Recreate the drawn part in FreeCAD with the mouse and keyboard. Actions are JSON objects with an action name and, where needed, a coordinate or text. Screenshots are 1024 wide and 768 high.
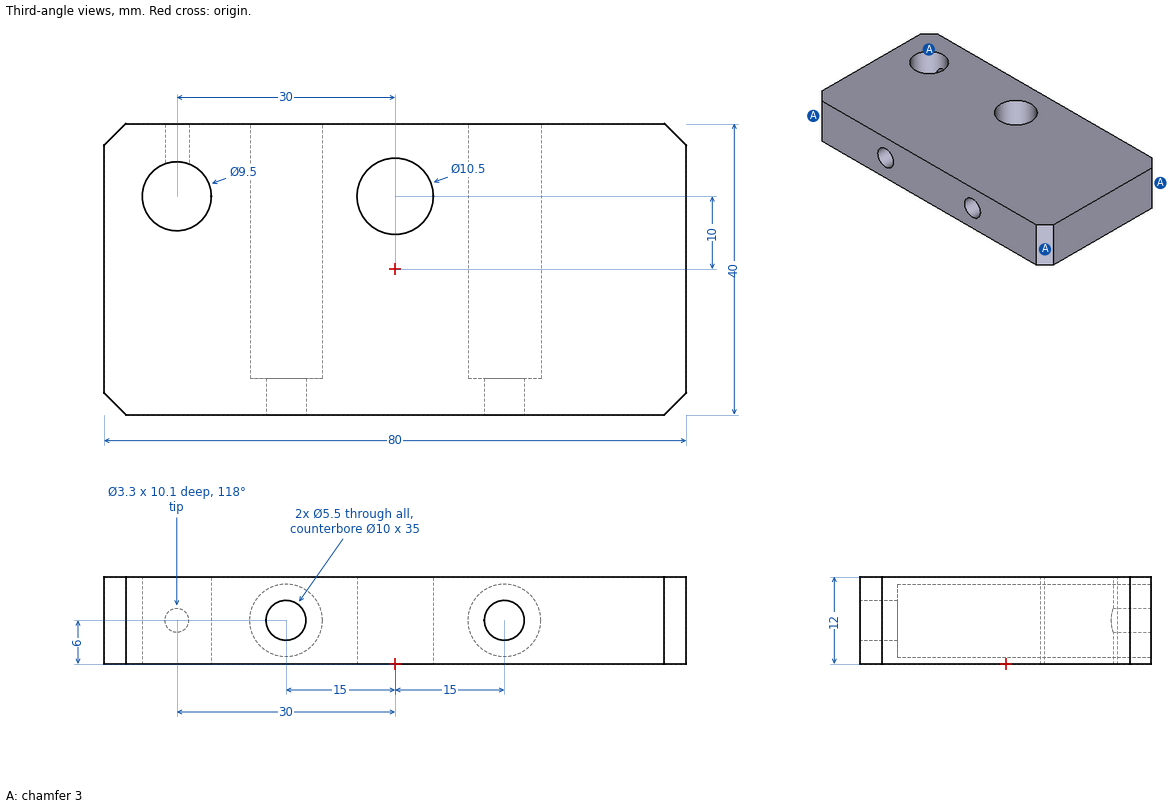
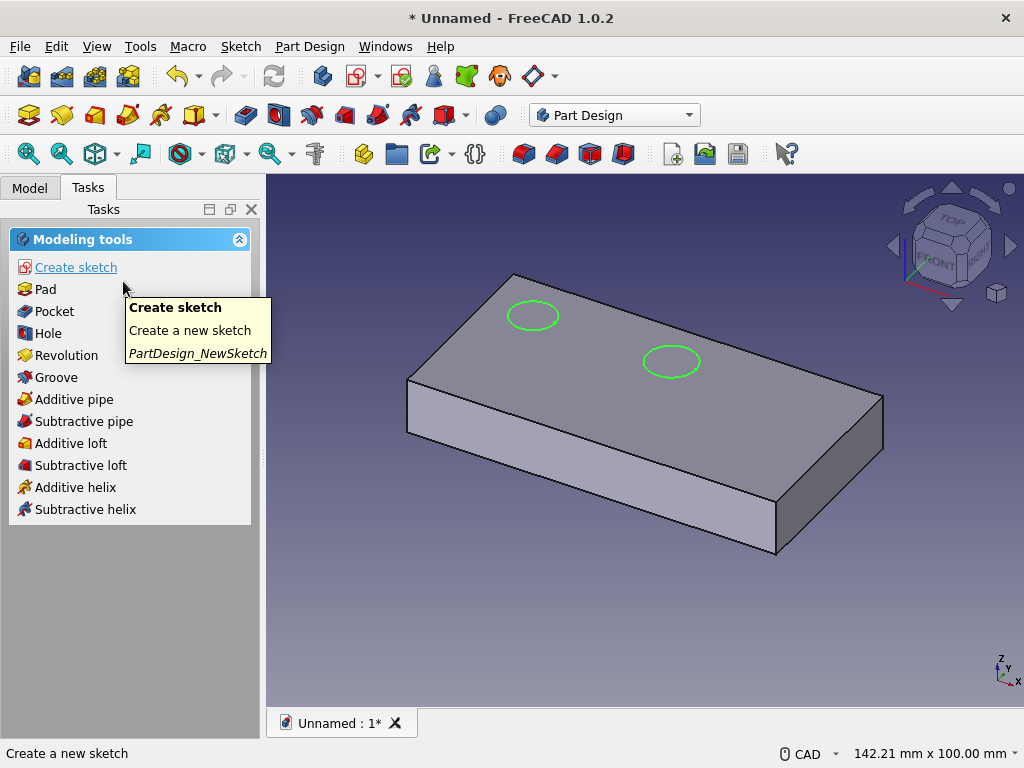
{"action": "left_click", "coordinate": [246, 116]}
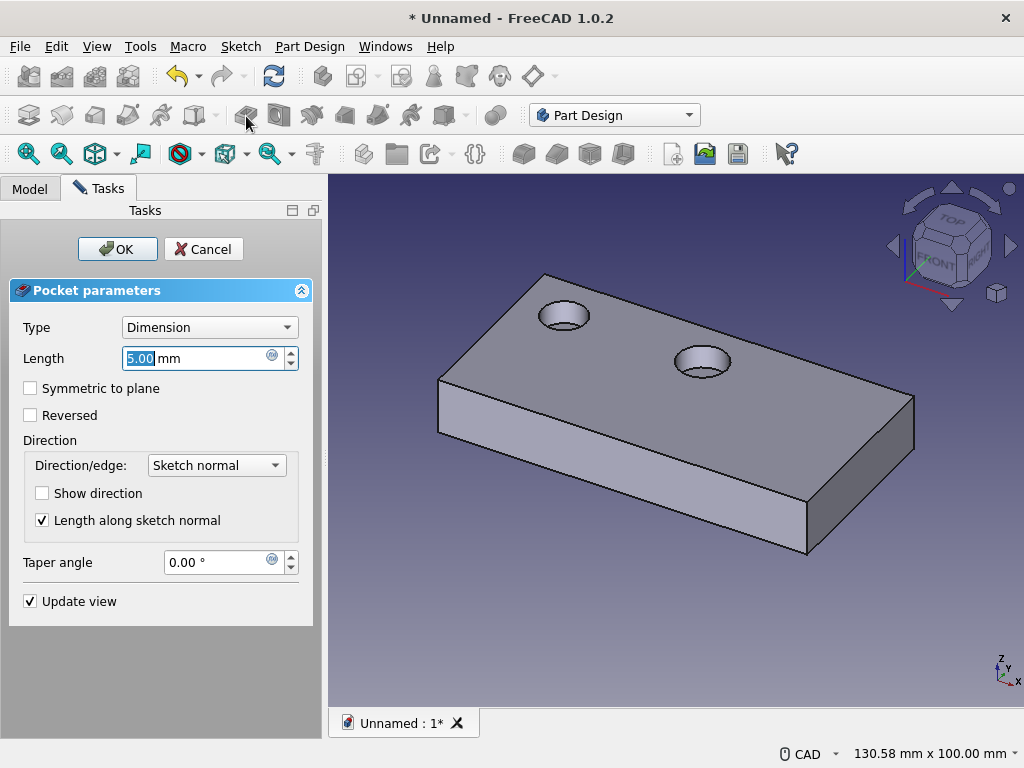
{"action": "left_click", "coordinate": [210, 328]}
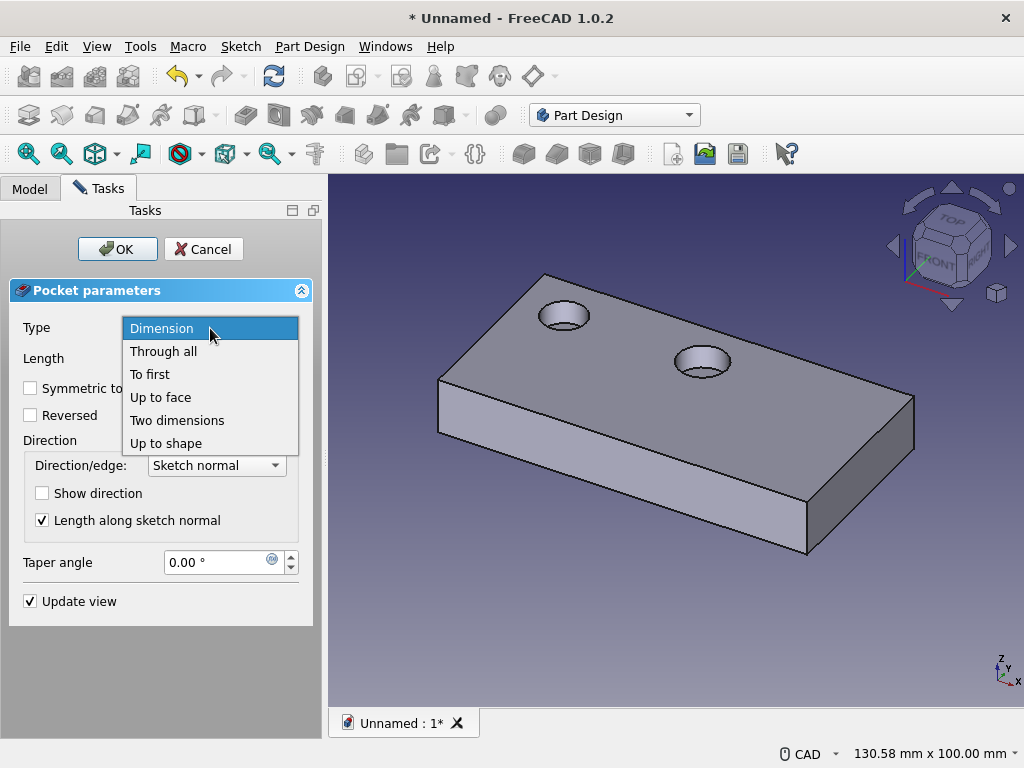
{"action": "left_click", "coordinate": [208, 352]}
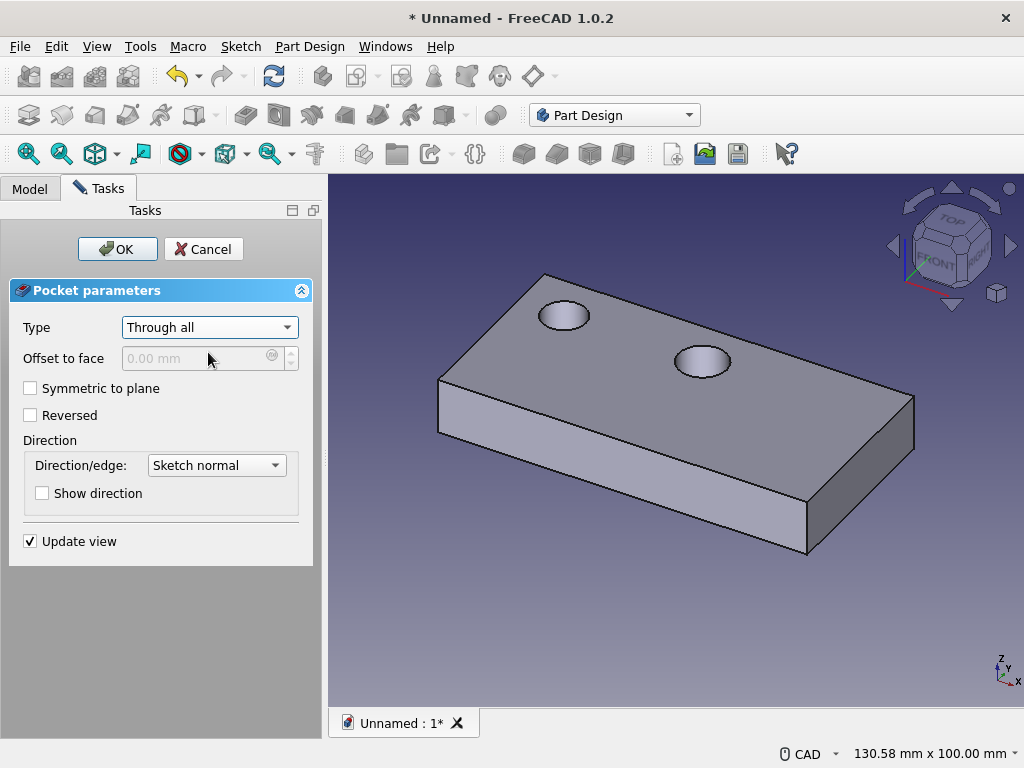
{"action": "left_click", "coordinate": [118, 249]}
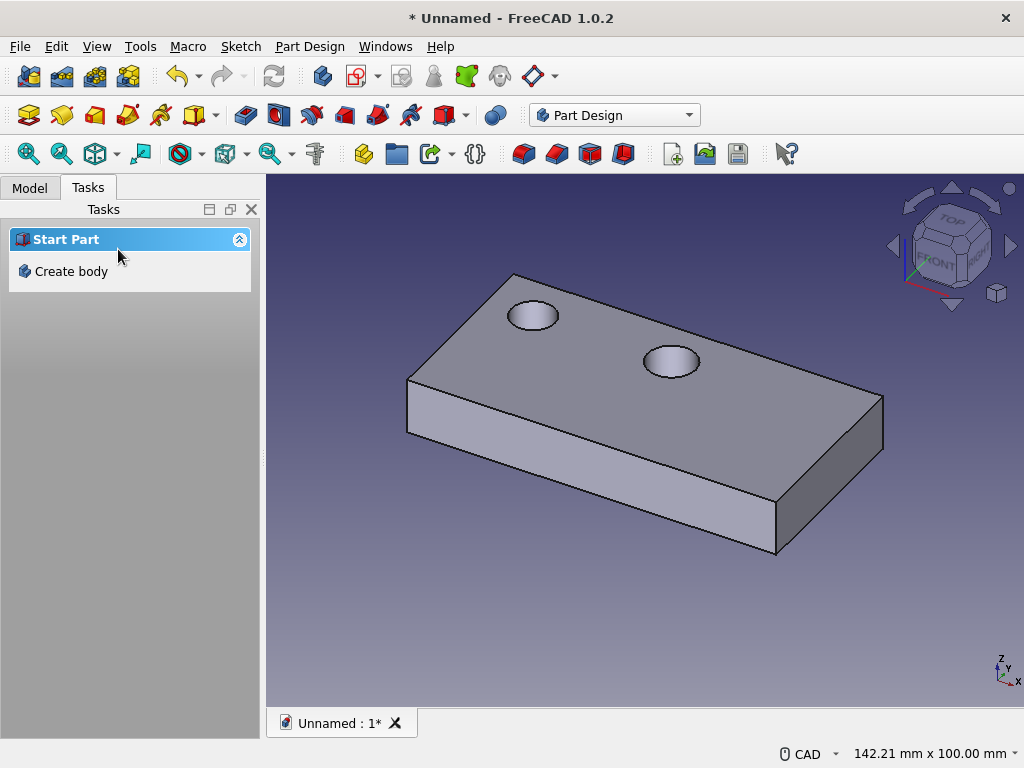
{"action": "key", "text": "4"}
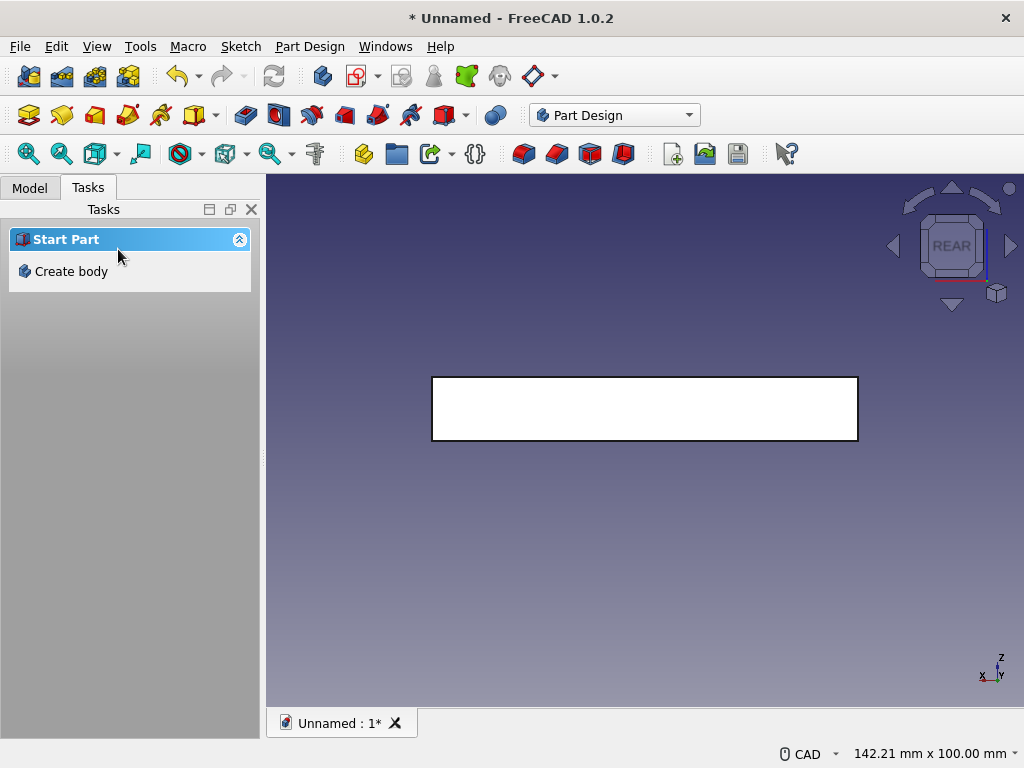
{"action": "left_click", "coordinate": [523, 408]}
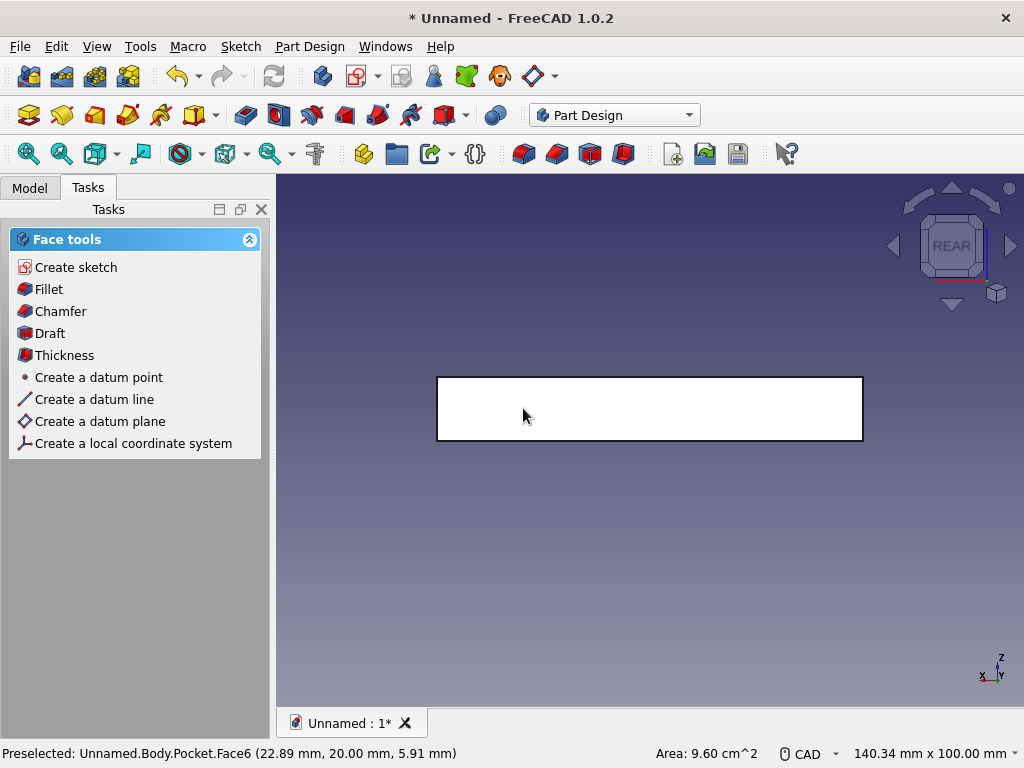
{"action": "left_click", "coordinate": [356, 76]}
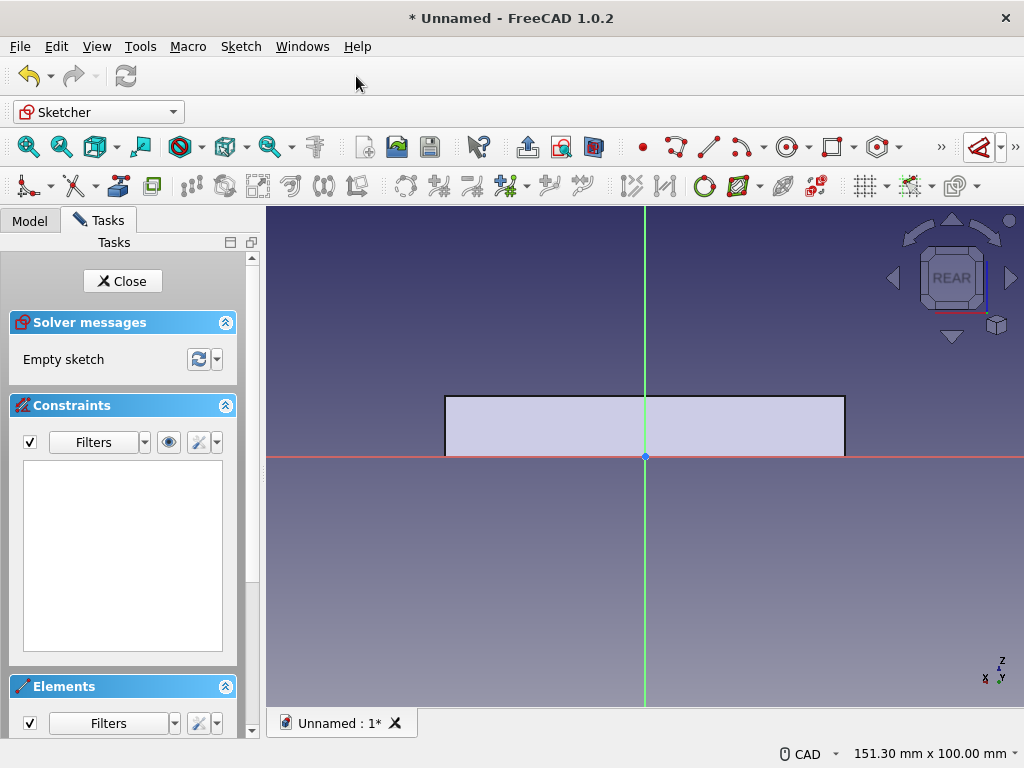
{"action": "scroll", "coordinate": [701, 417], "scroll_direction": "up", "scroll_amount": 4}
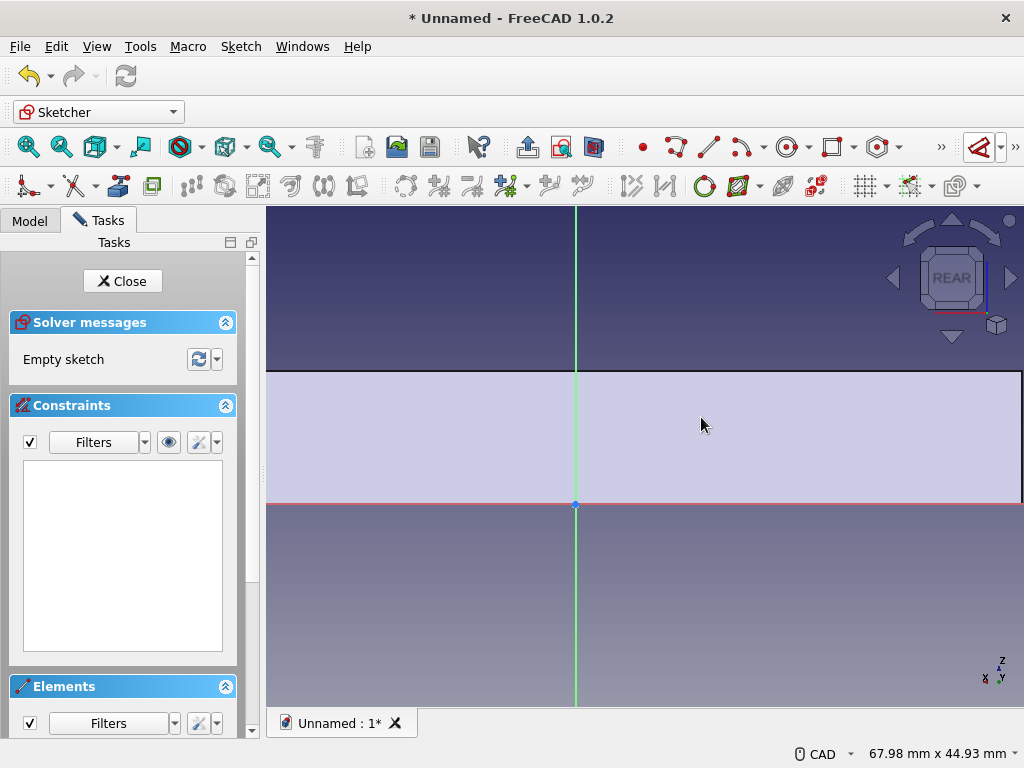
{"action": "key", "text": "g c"}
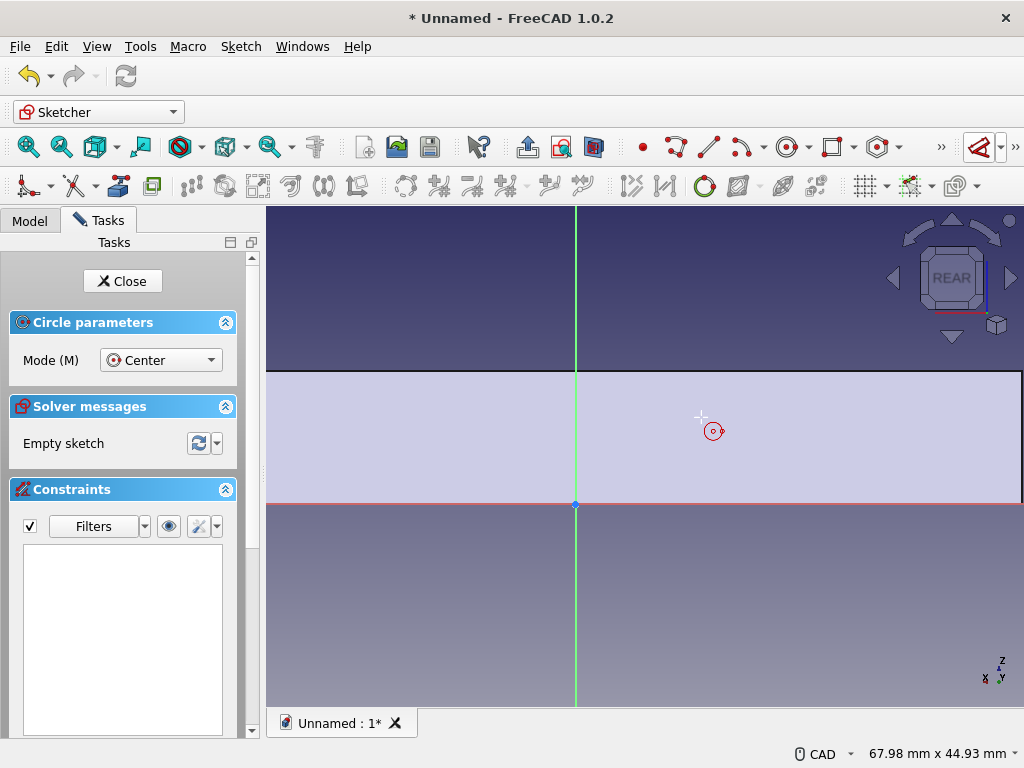
{"action": "left_click", "coordinate": [743, 437]}
{"action": "left_click", "coordinate": [765, 416]}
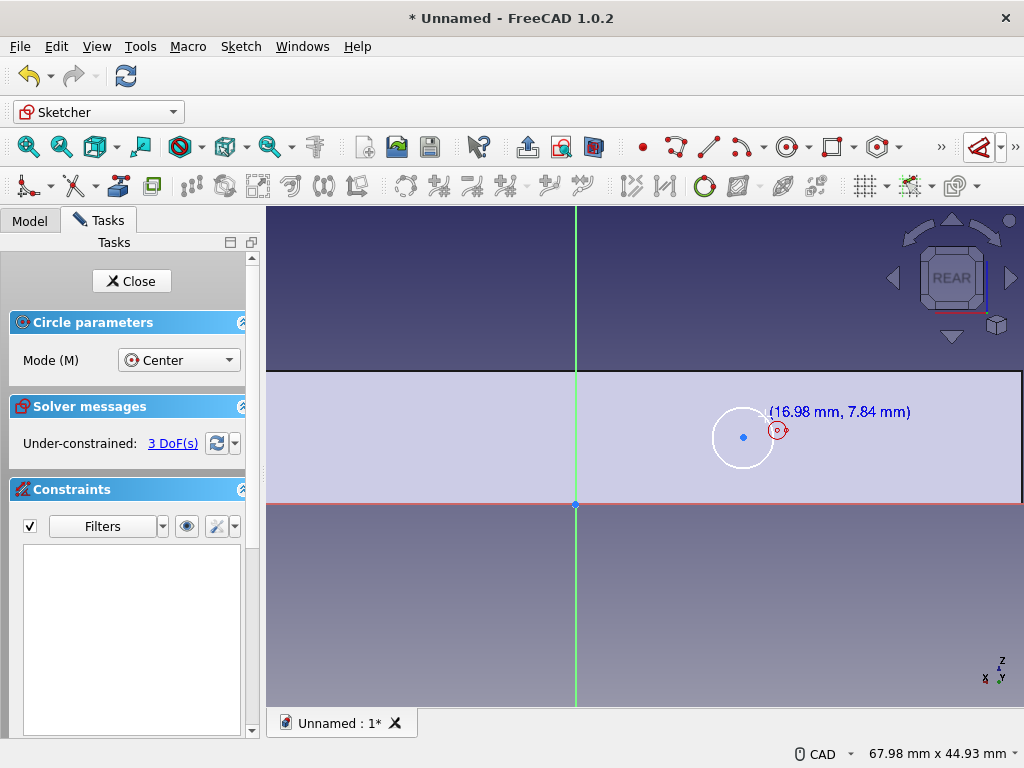
{"action": "left_click", "coordinate": [408, 437]}
{"action": "left_click", "coordinate": [430, 416]}
{"action": "key", "text": "Escape"}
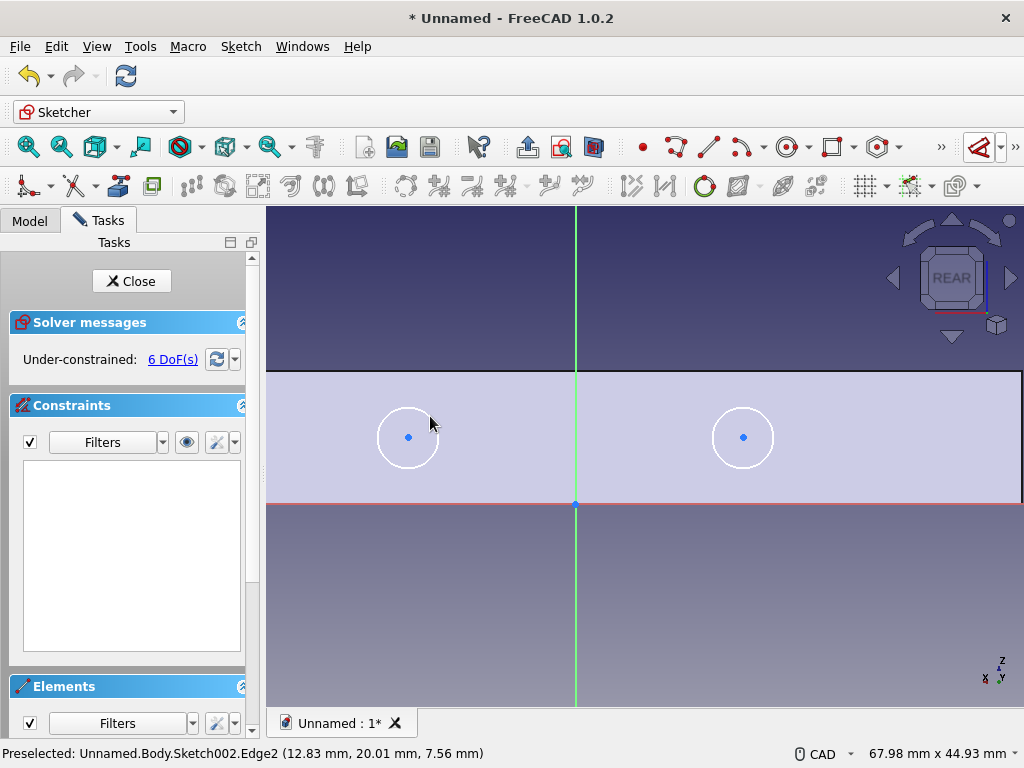
{"action": "left_click", "coordinate": [764, 416]}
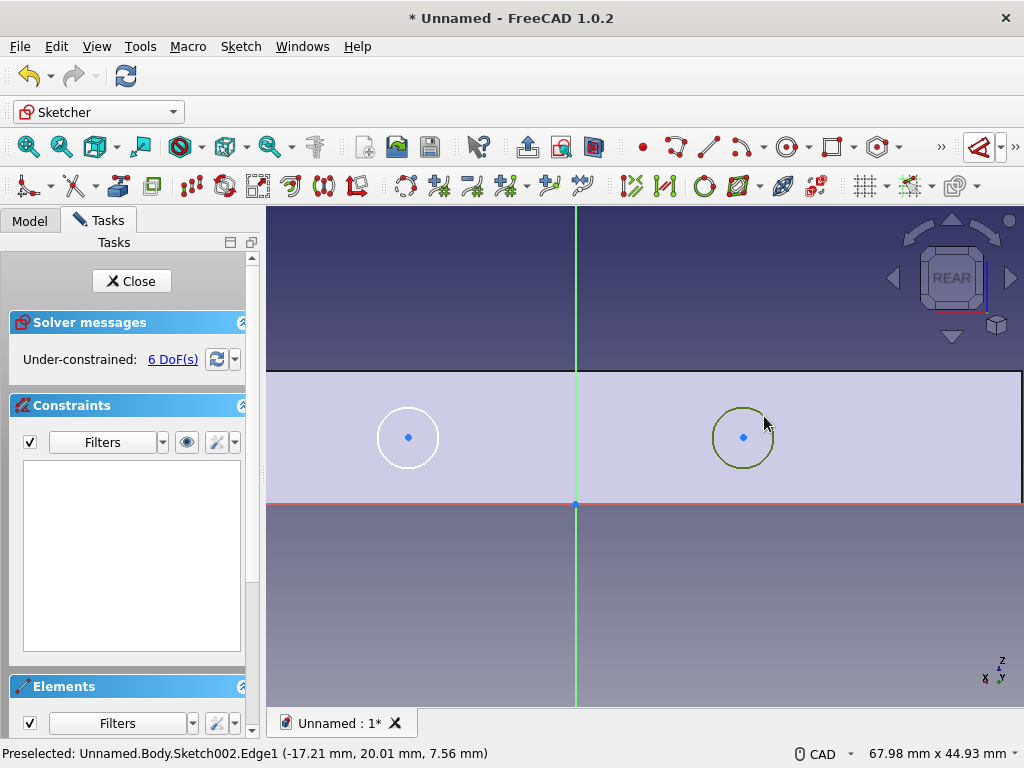
{"action": "left_click", "coordinate": [429, 416]}